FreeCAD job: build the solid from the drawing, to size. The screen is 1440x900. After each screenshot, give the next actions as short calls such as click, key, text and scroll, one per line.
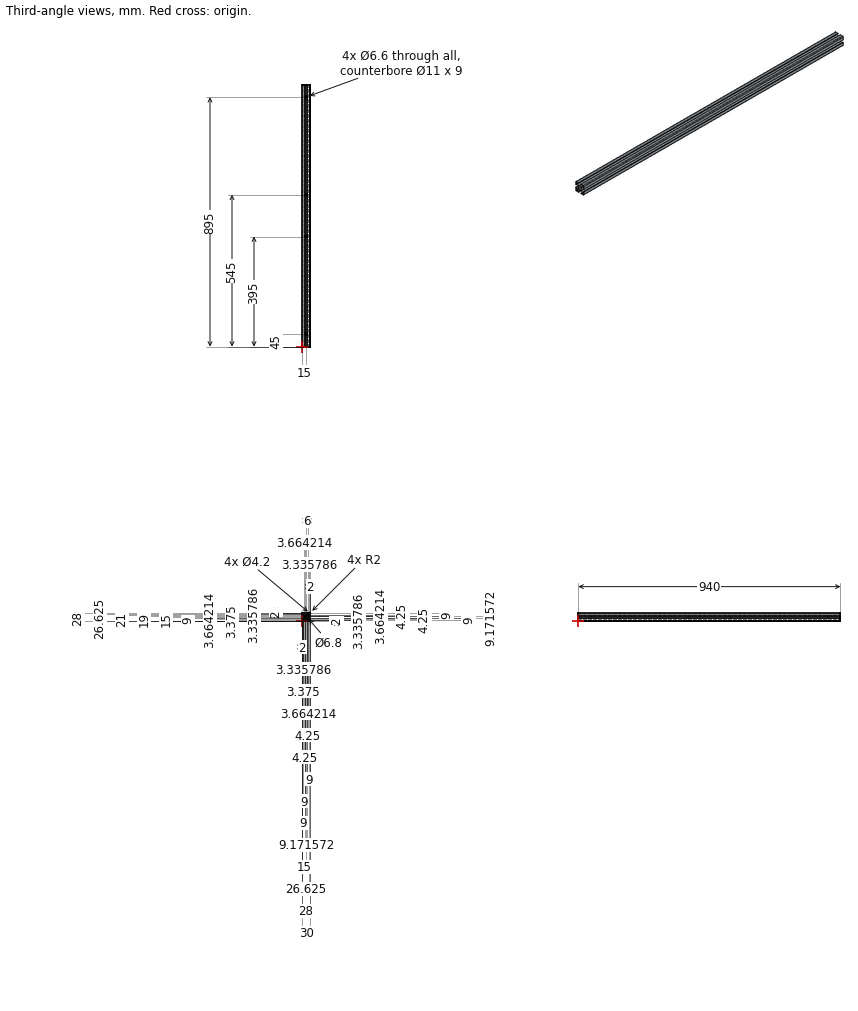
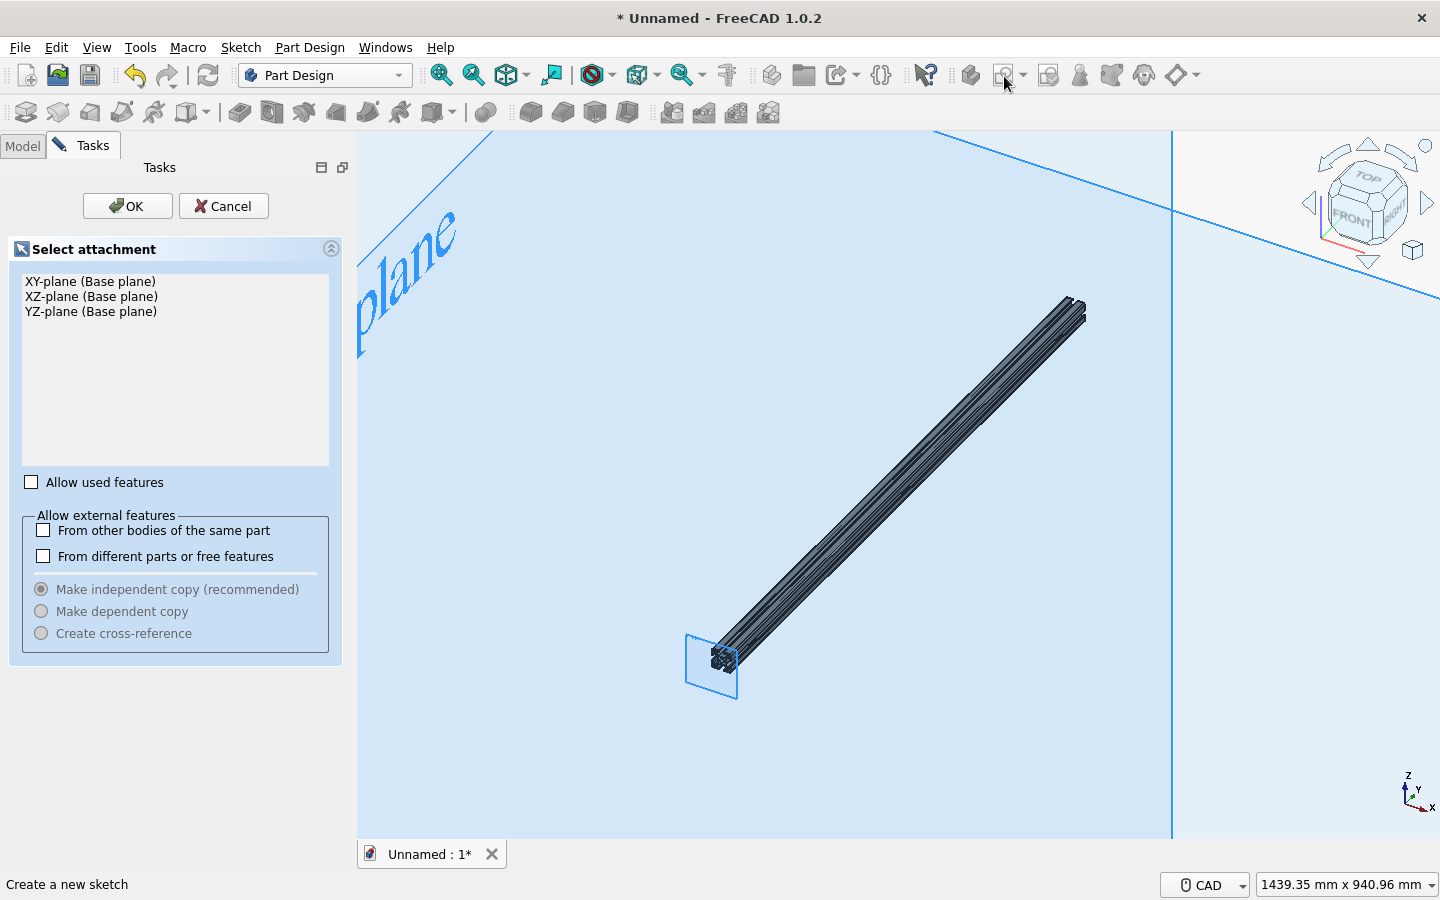
click(82, 282)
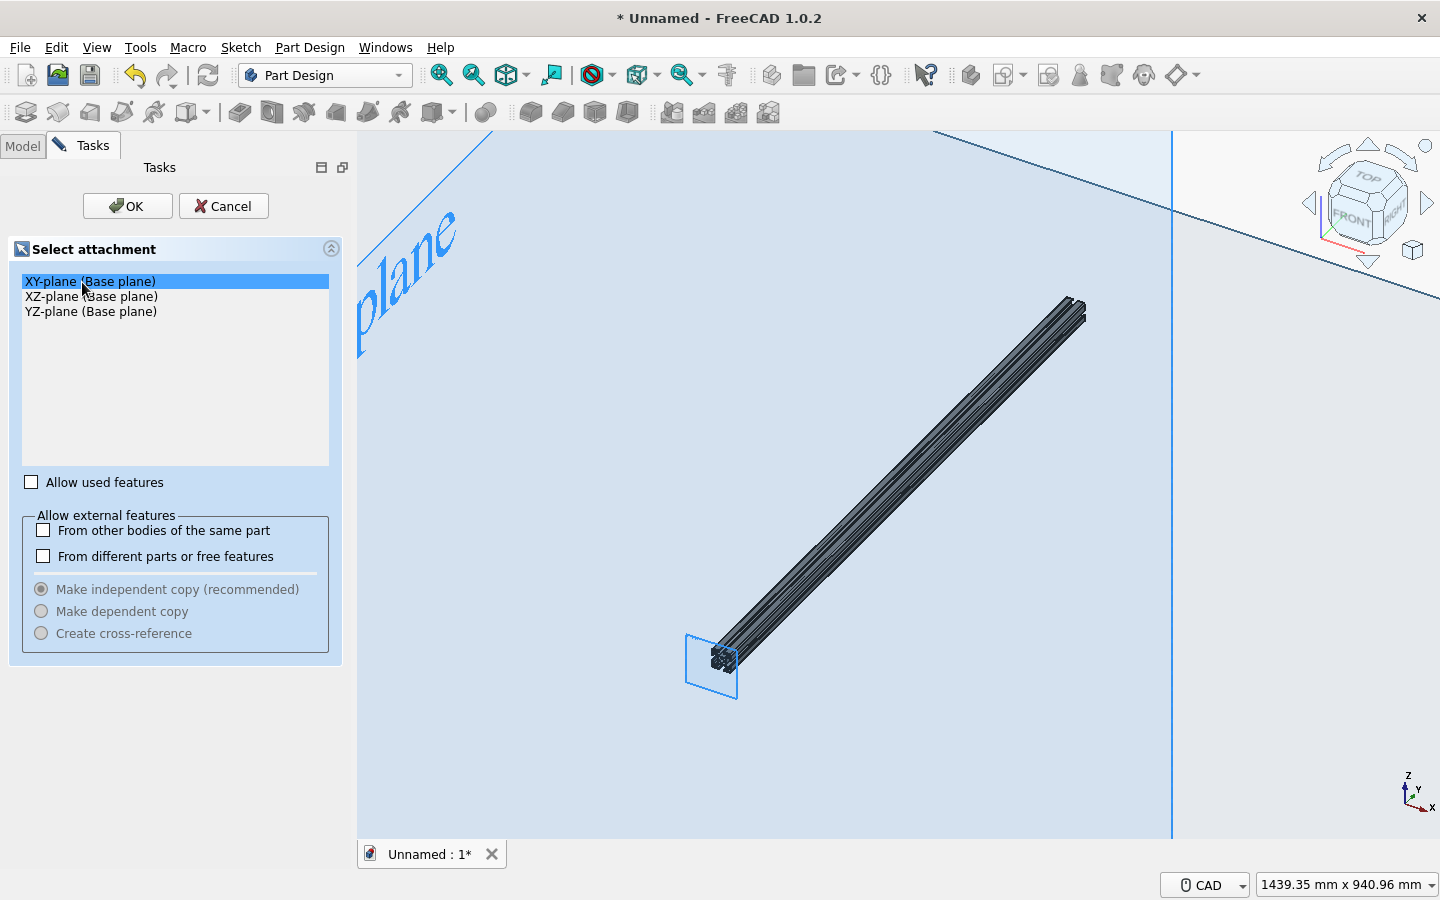
click(128, 206)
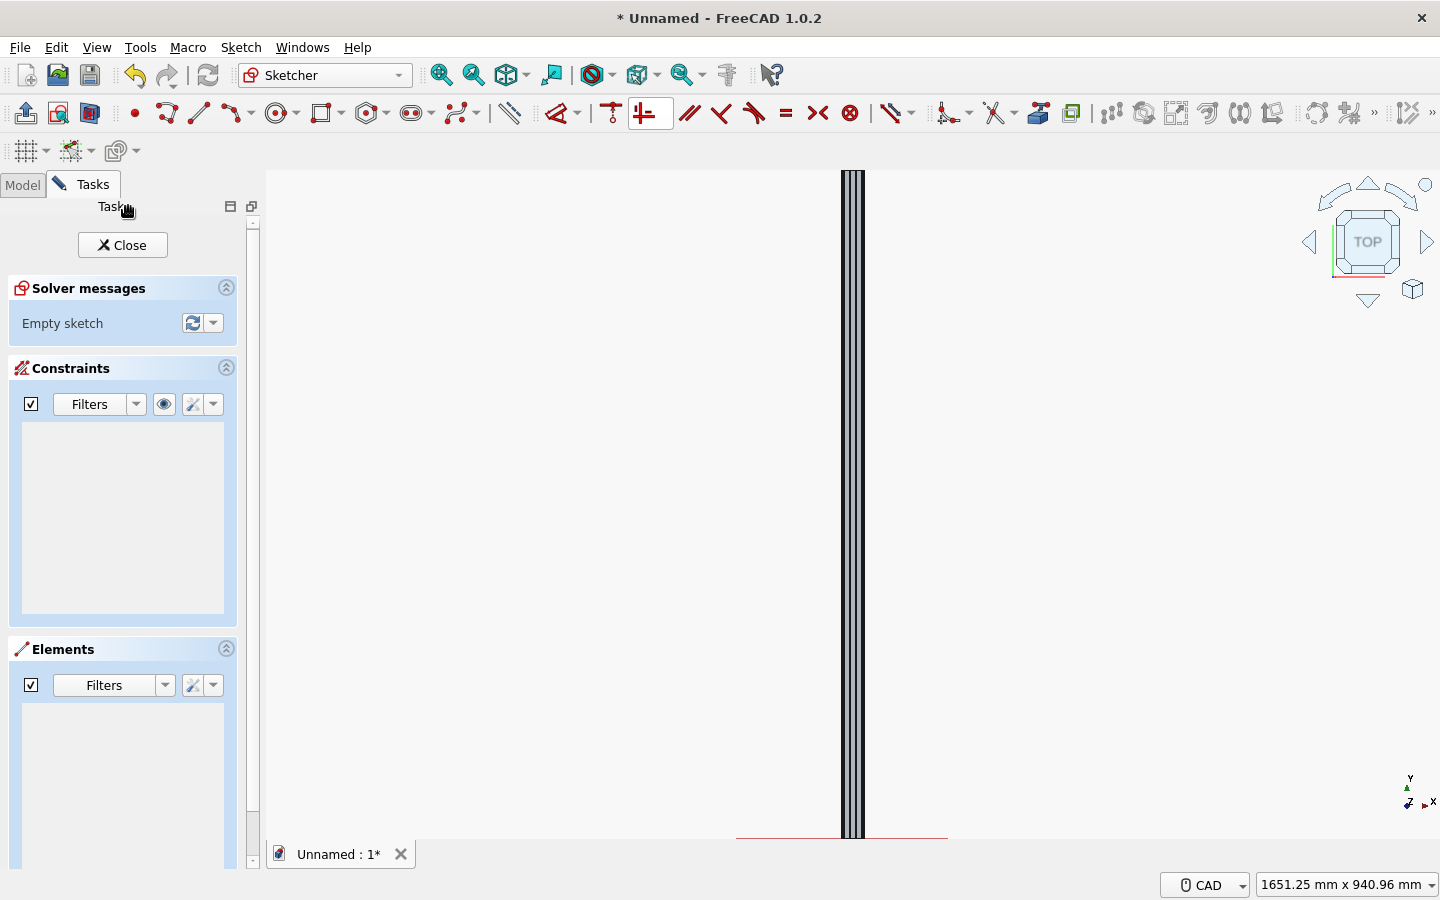
click(90, 114)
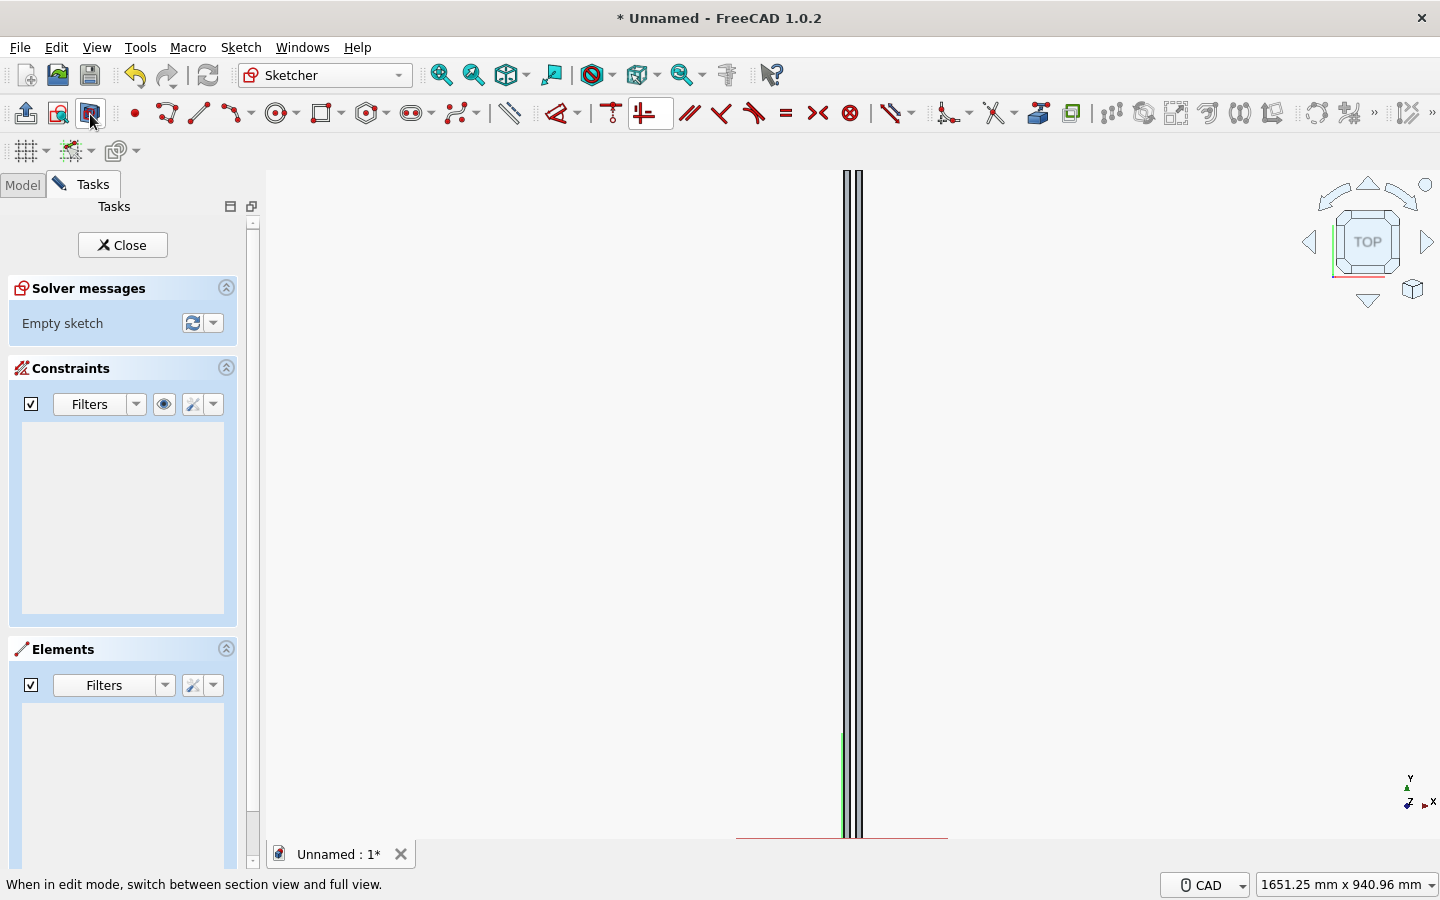
scroll(654, 474, down, 2)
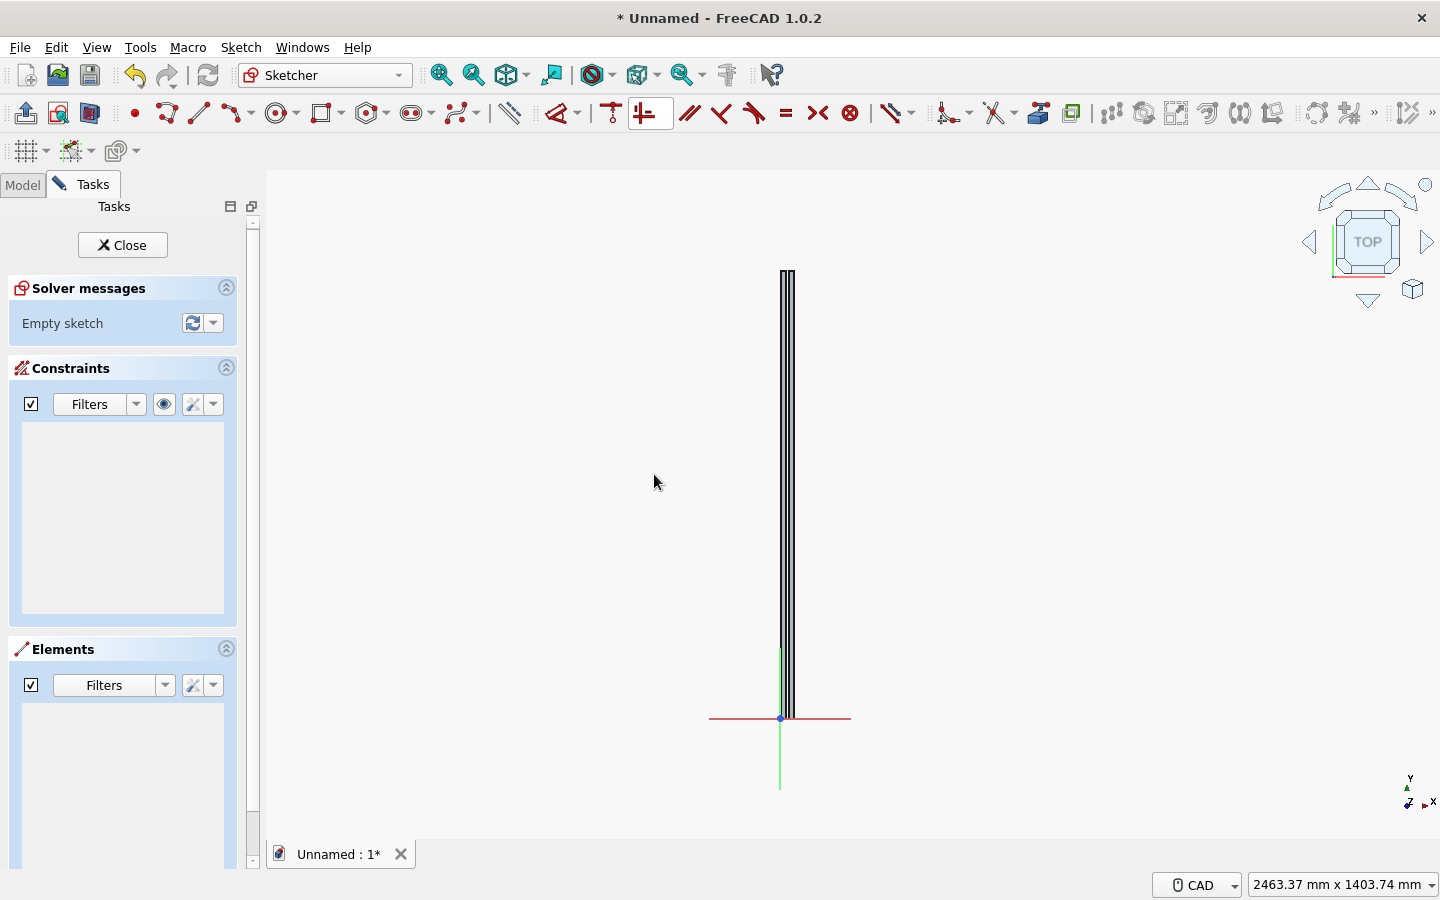
click(276, 114)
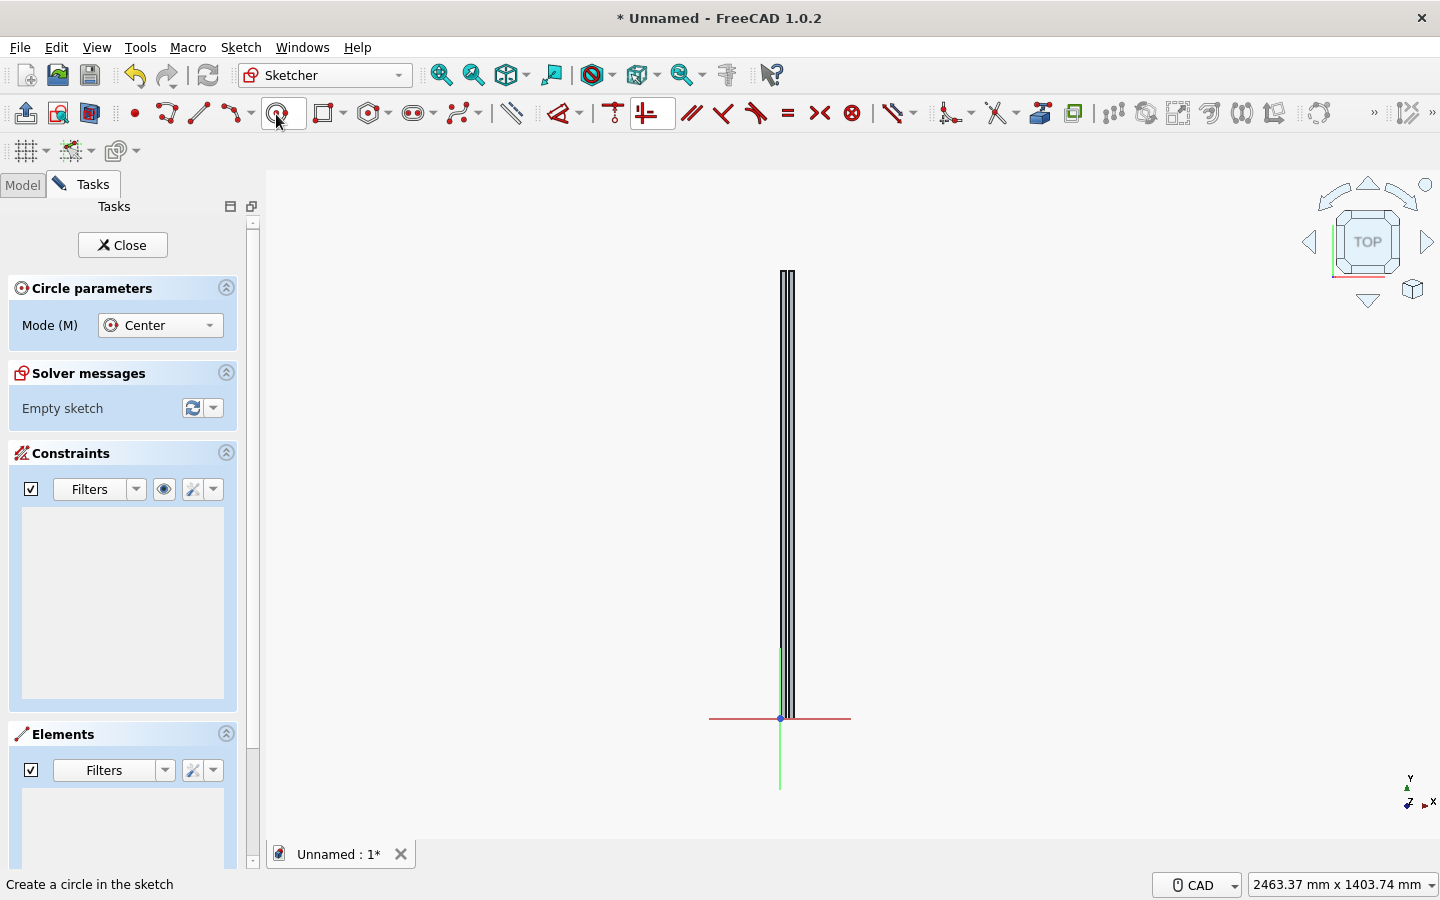
scroll(788, 292, up, 14)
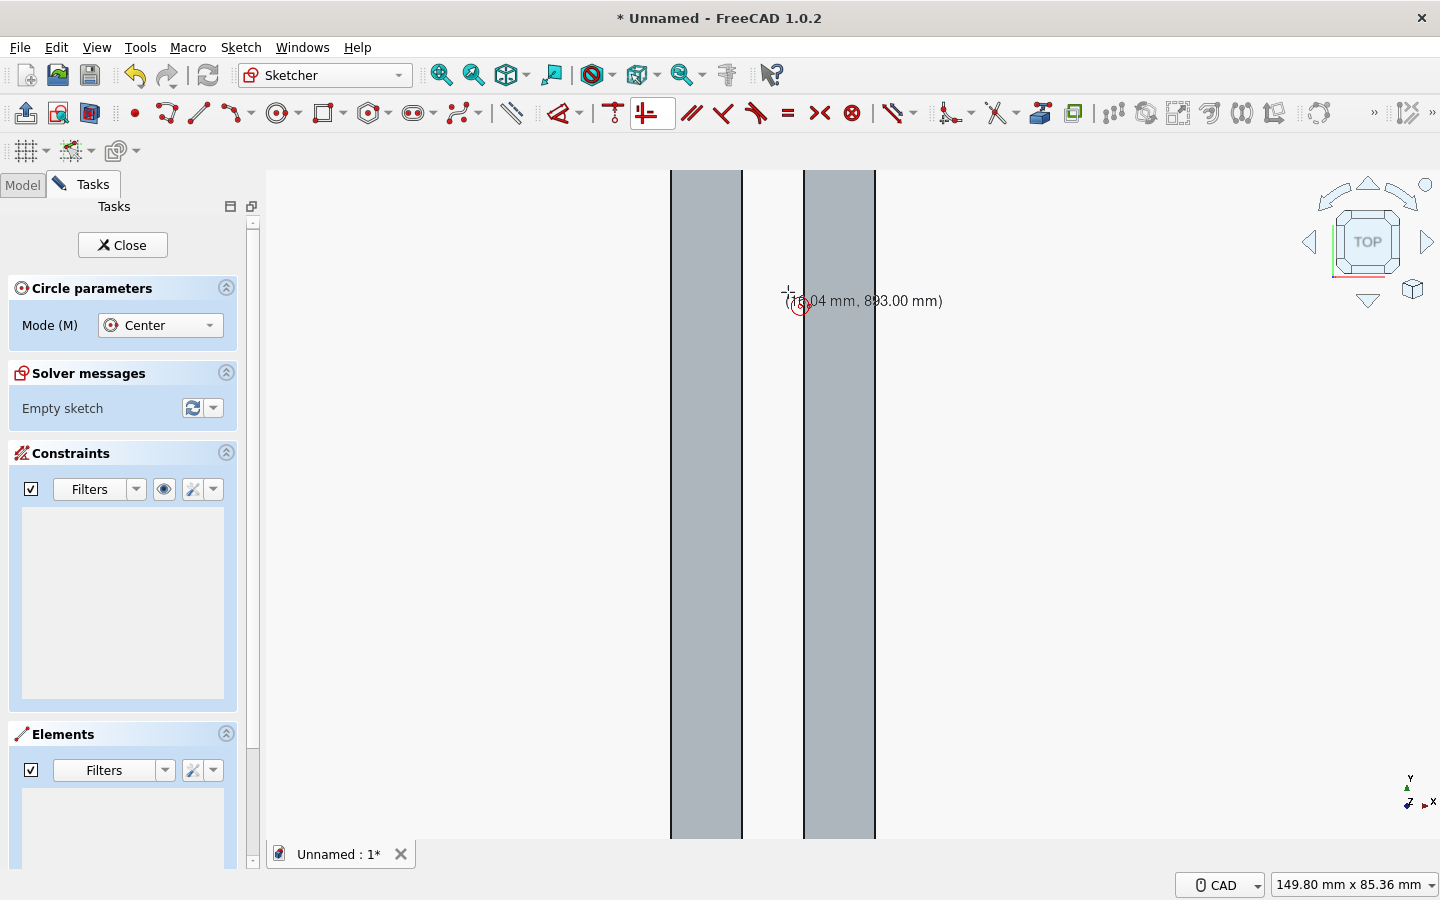
scroll(788, 292, down, 14)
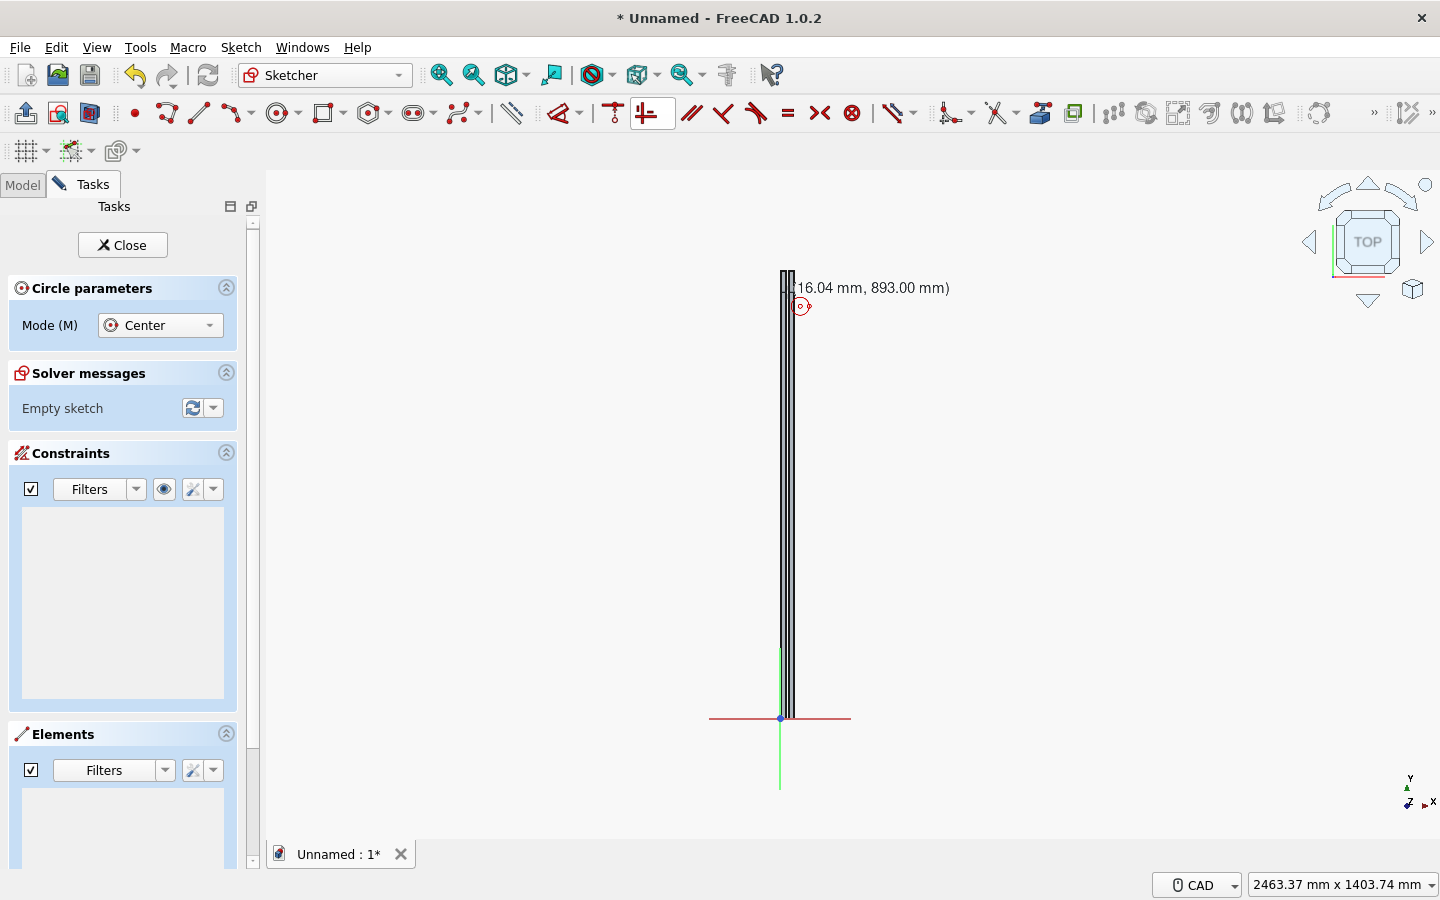
scroll(788, 292, up, 4)